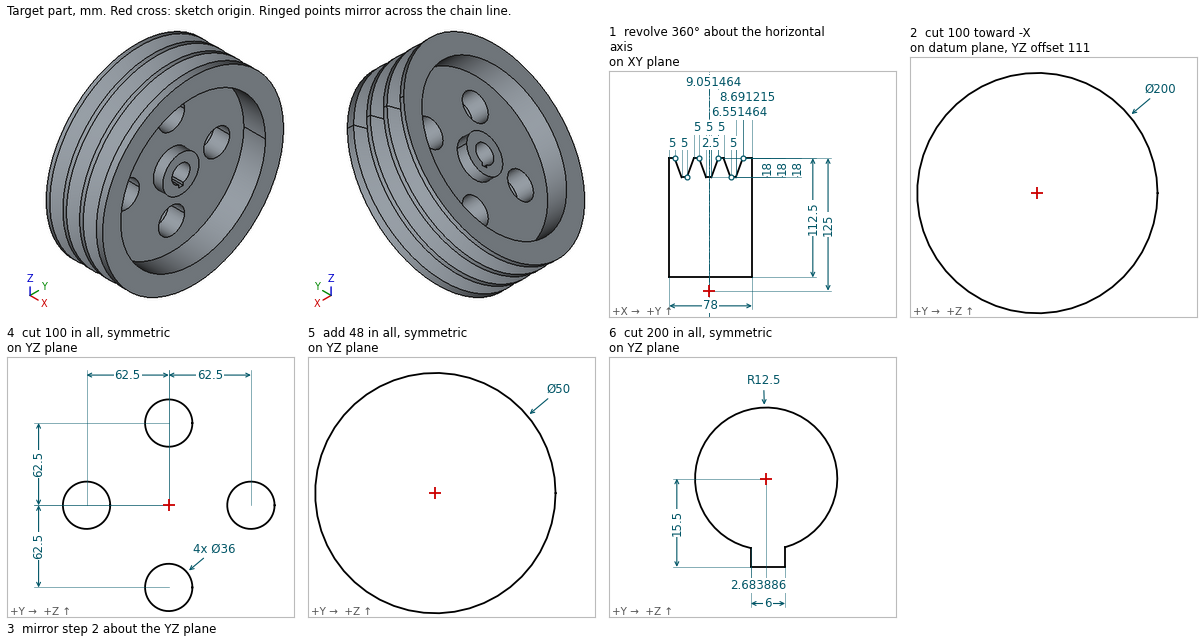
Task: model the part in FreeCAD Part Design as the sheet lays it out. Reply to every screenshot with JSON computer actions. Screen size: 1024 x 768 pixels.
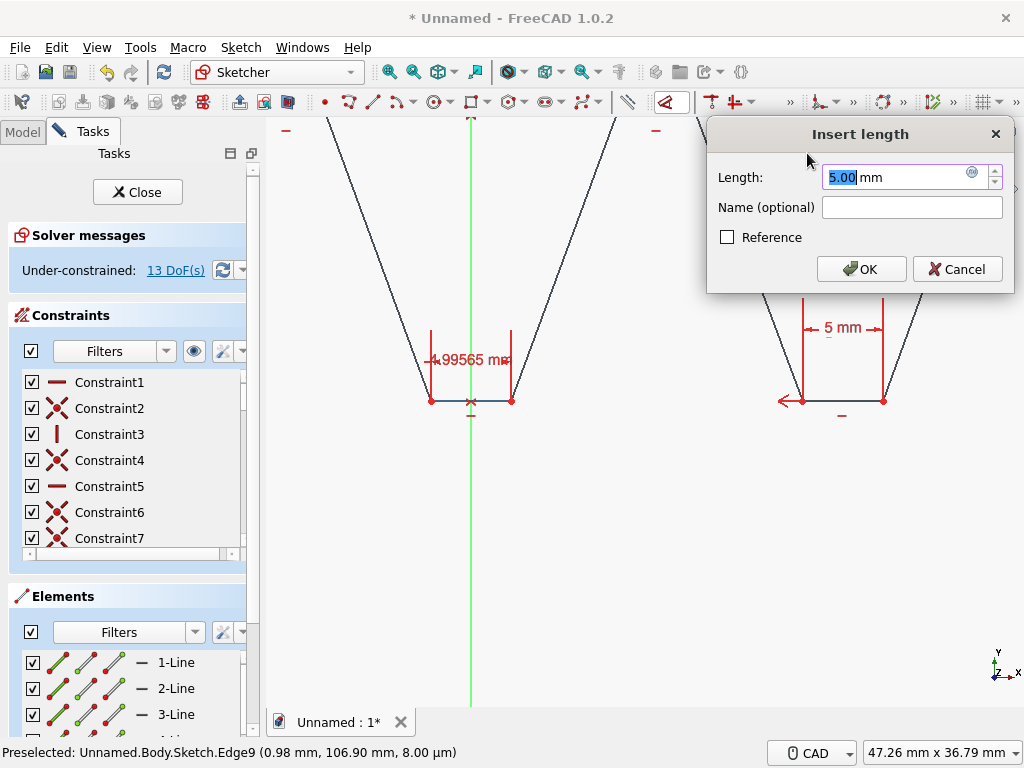
{"action": "type", "text": "5"}
{"action": "key", "text": "Return"}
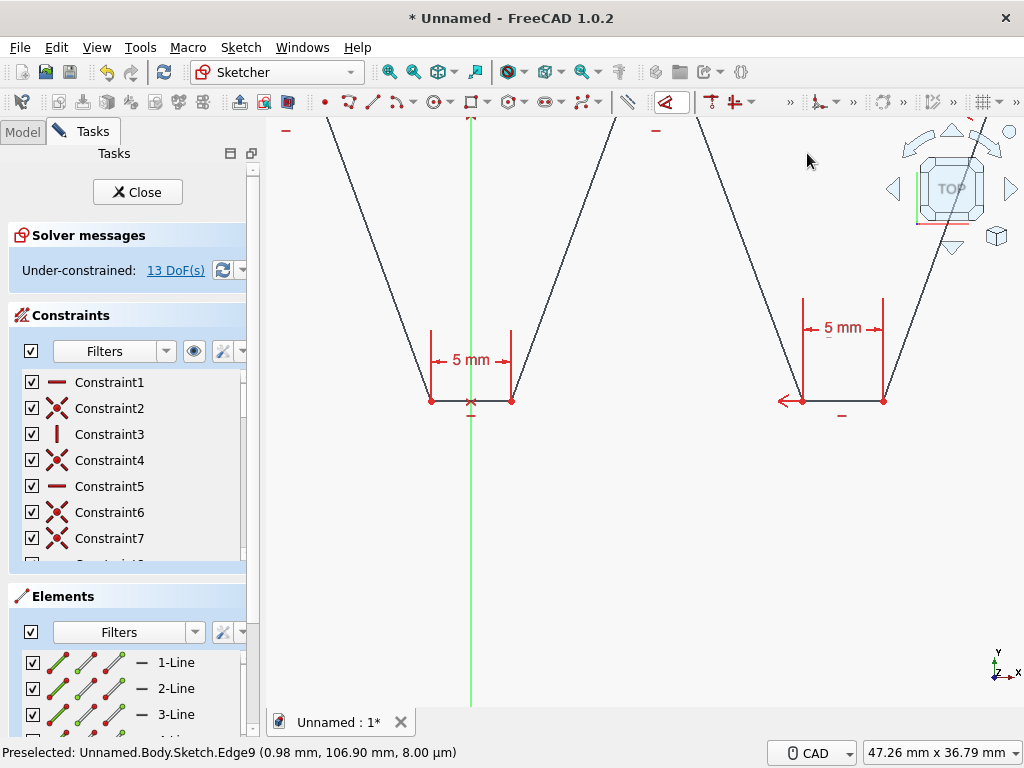
{"action": "scroll", "coordinate": [596, 235], "scroll_direction": "down", "scroll_amount": 8}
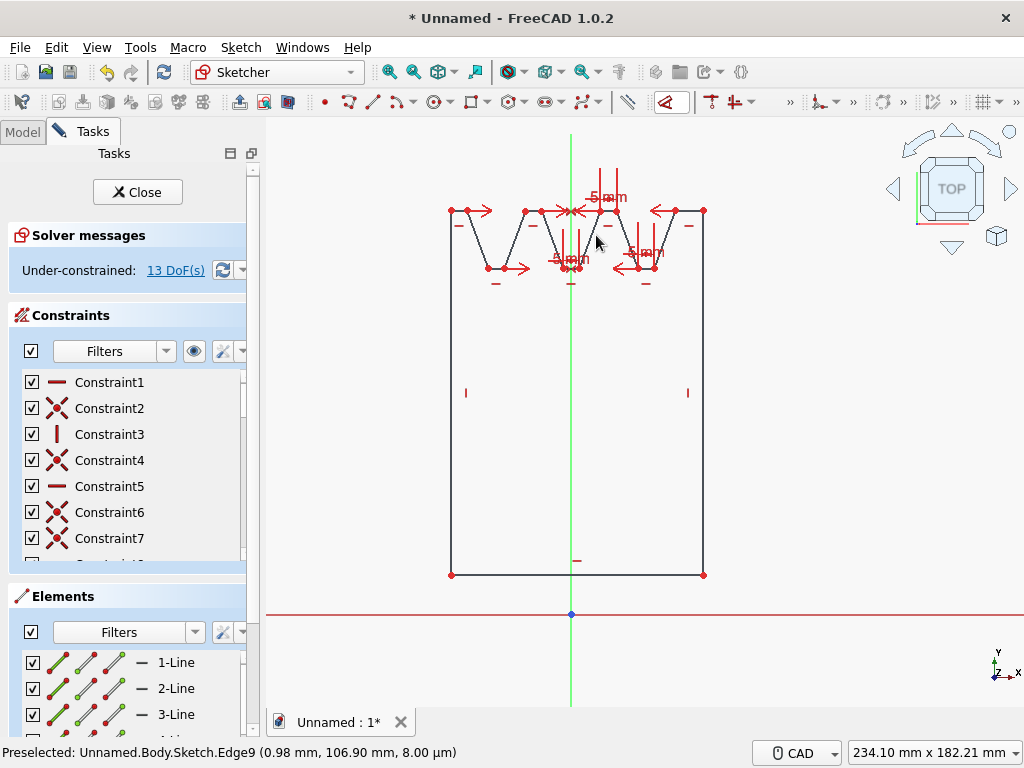
{"action": "scroll", "coordinate": [537, 211], "scroll_direction": "up", "scroll_amount": 6}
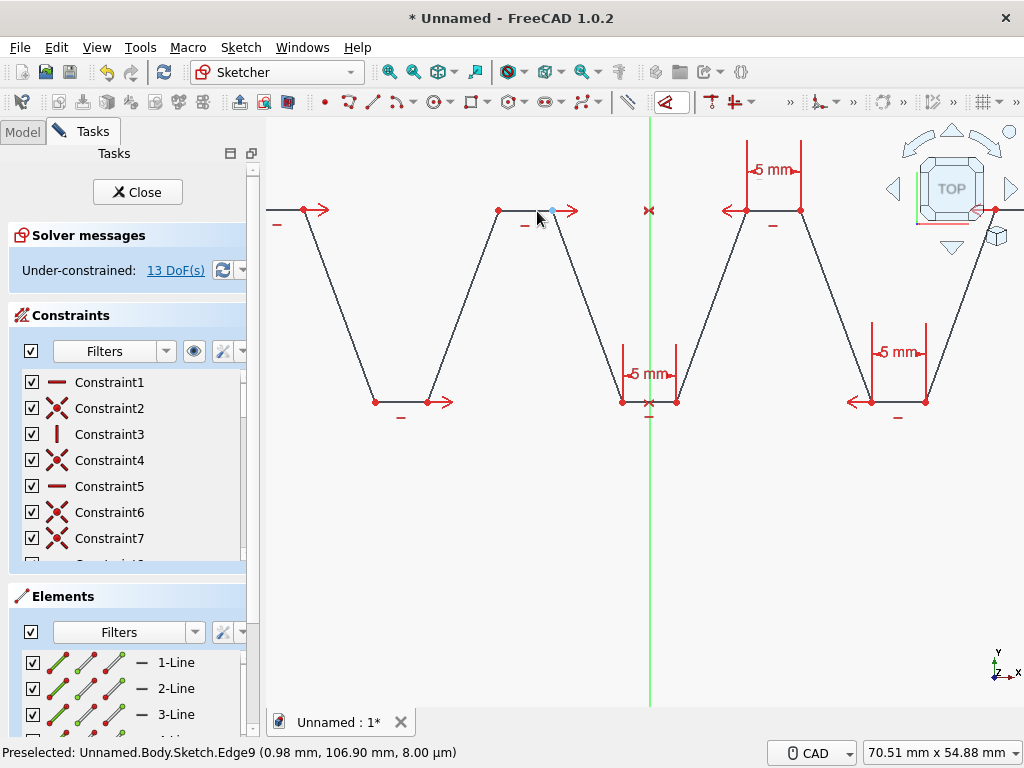
{"action": "left_click", "coordinate": [536, 211]}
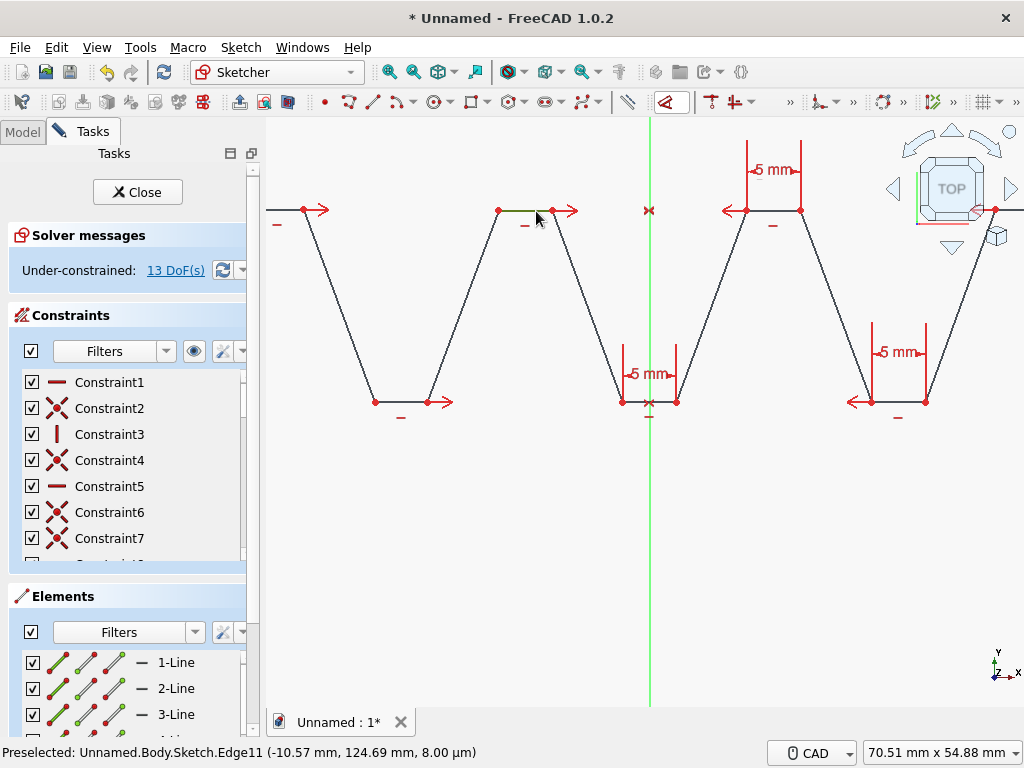
{"action": "left_click", "coordinate": [684, 102]}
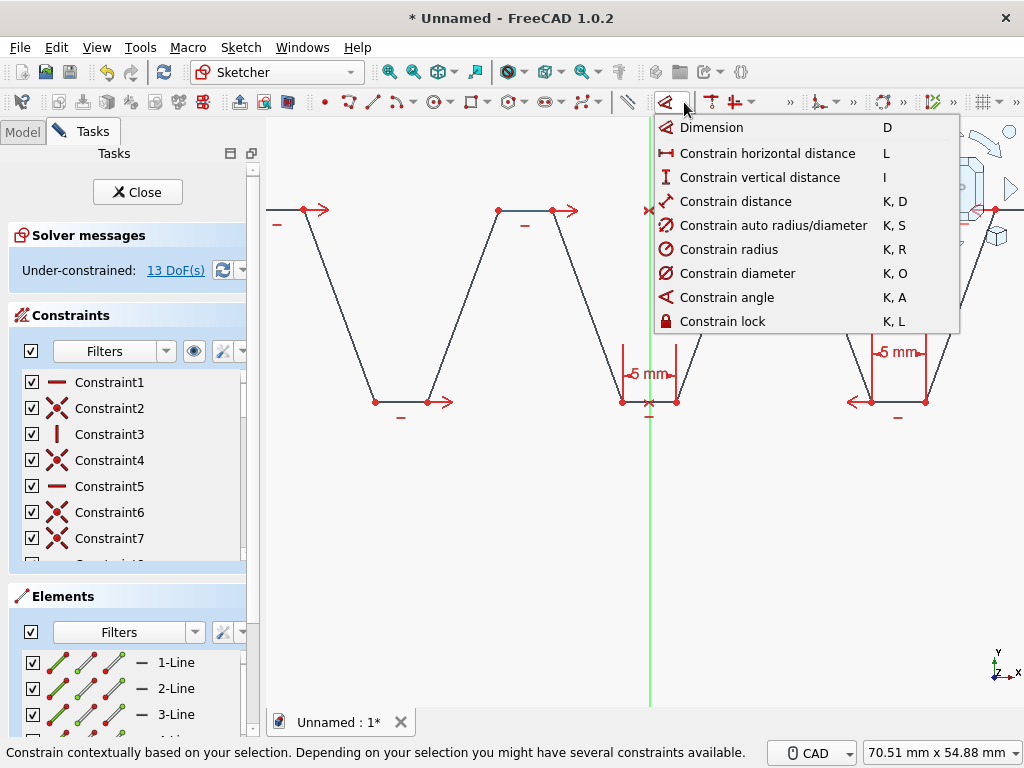
{"action": "left_click", "coordinate": [807, 153]}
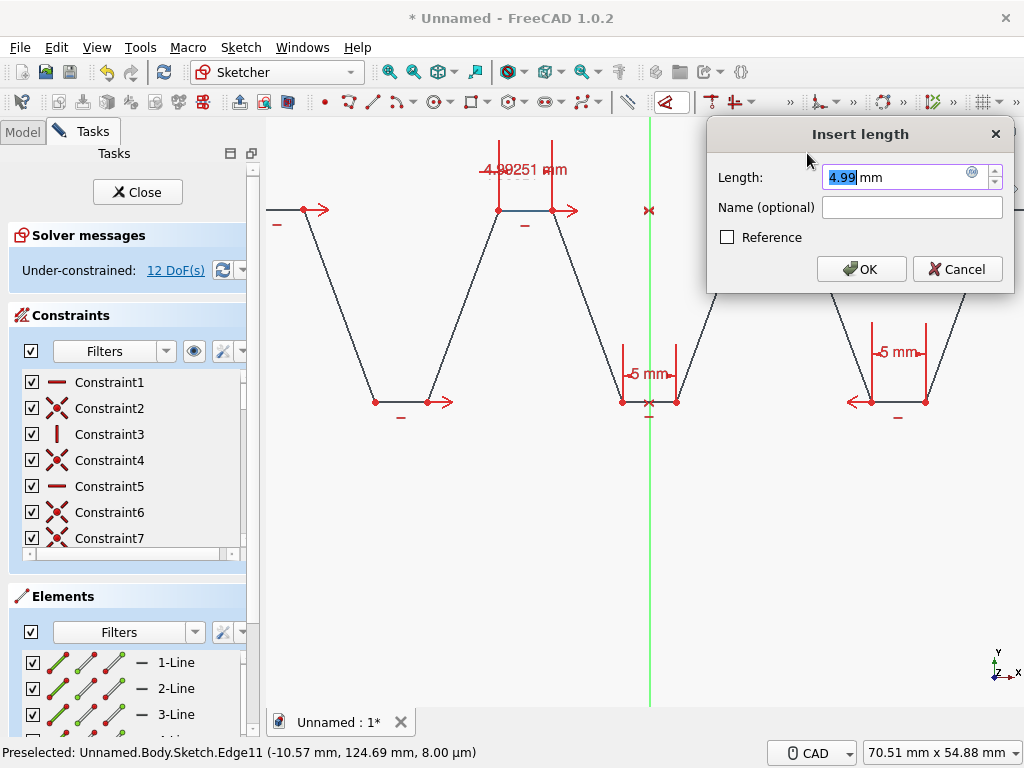
{"action": "type", "text": "5"}
{"action": "key", "text": "Return"}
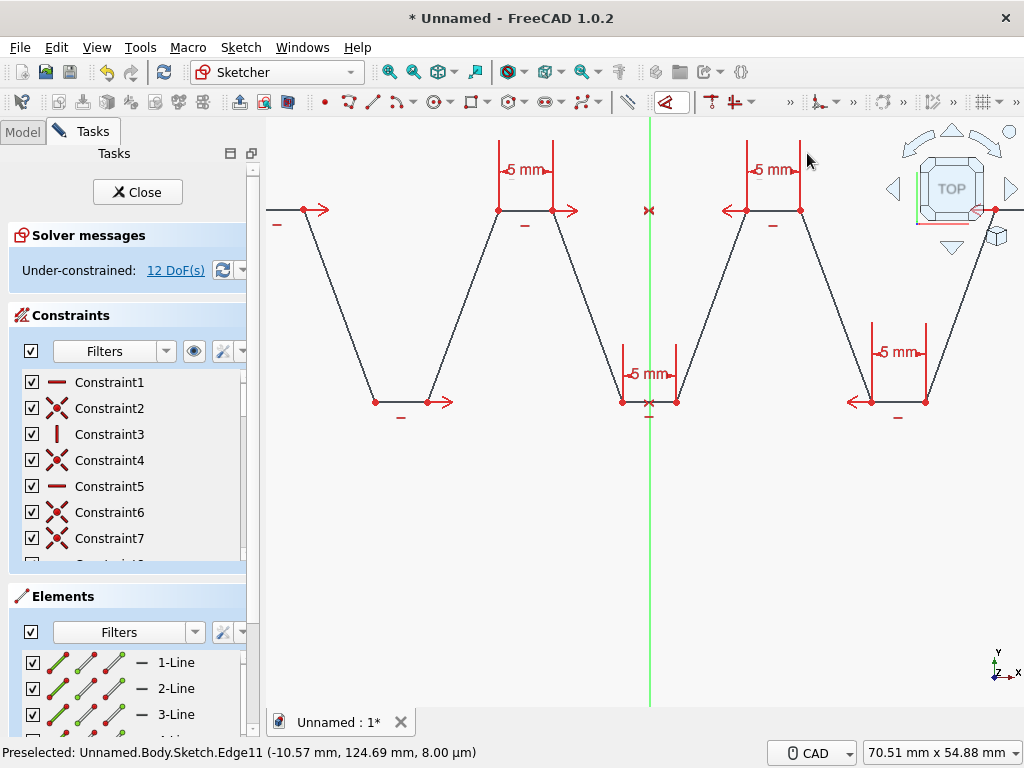
{"action": "left_click", "coordinate": [412, 402]}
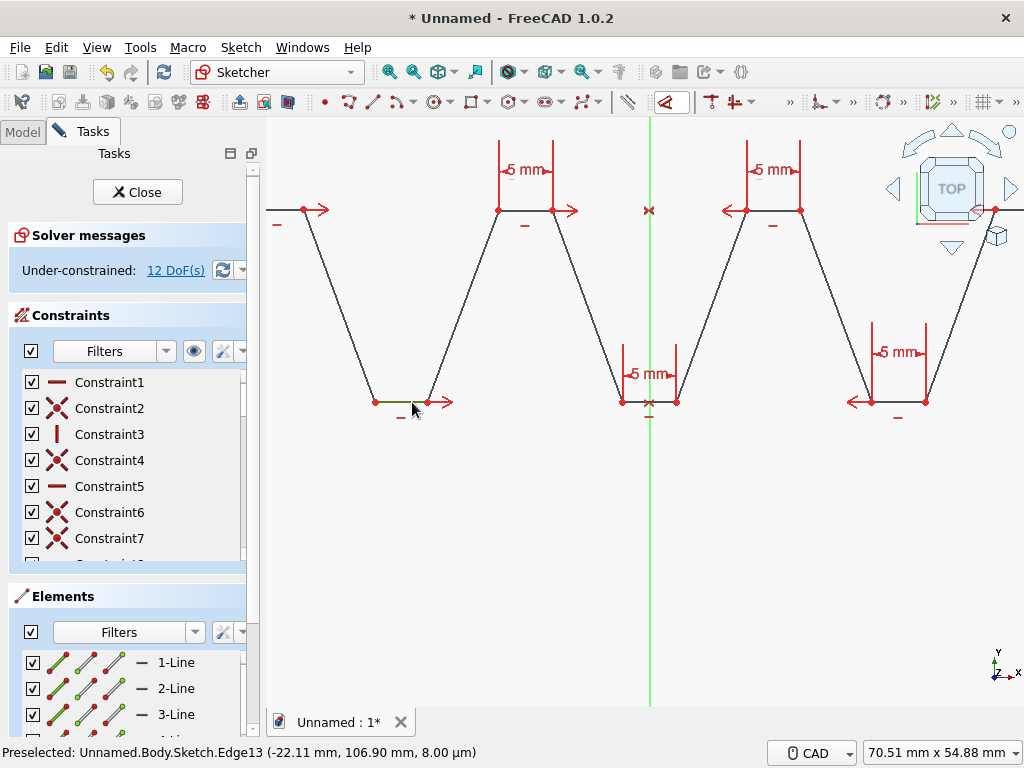
{"action": "key", "text": "l"}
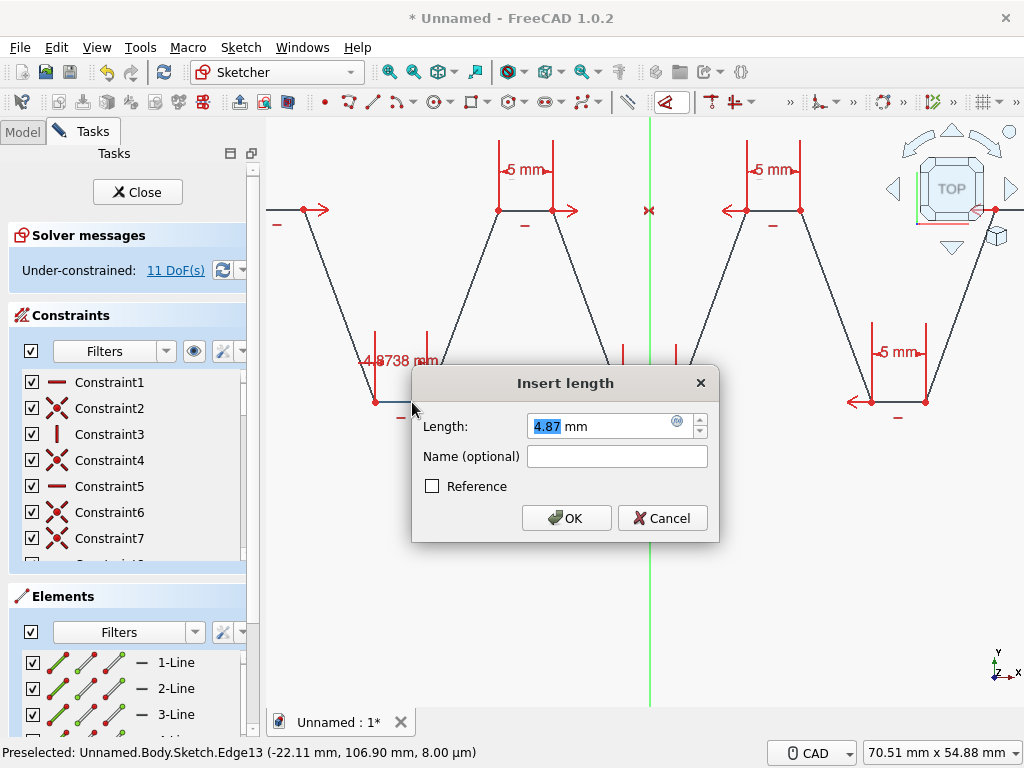
{"action": "type", "text": "5"}
{"action": "key", "text": "Return"}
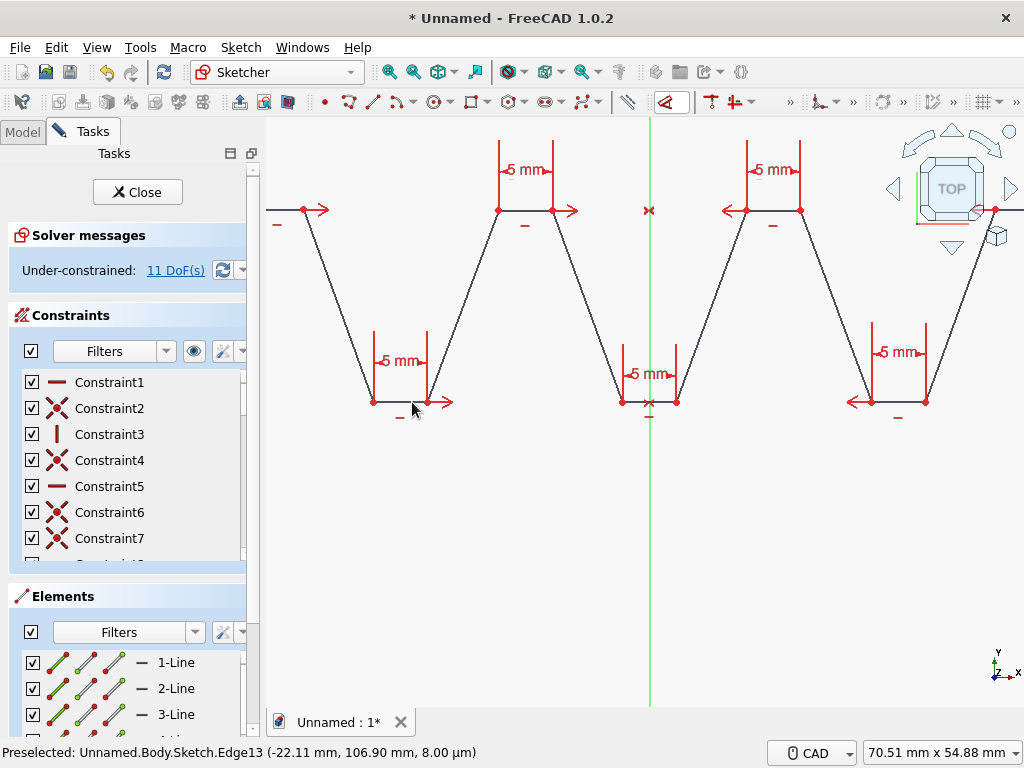
{"action": "scroll", "coordinate": [536, 210], "scroll_direction": "down", "scroll_amount": 6}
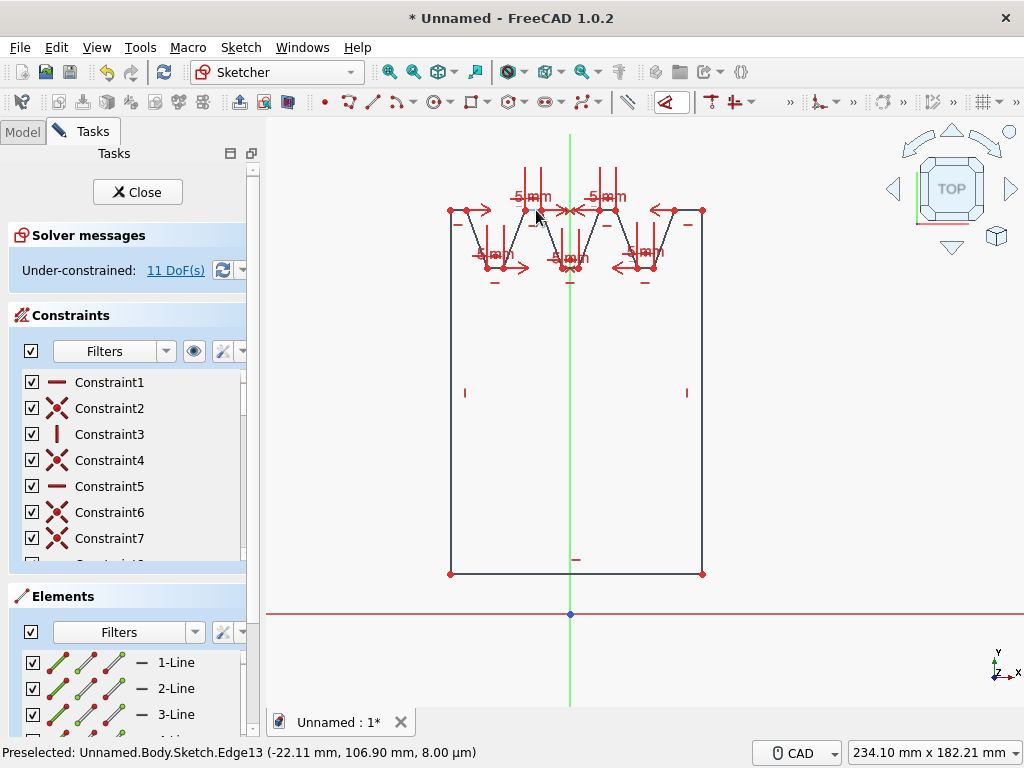
{"action": "scroll", "coordinate": [462, 210], "scroll_direction": "up", "scroll_amount": 6}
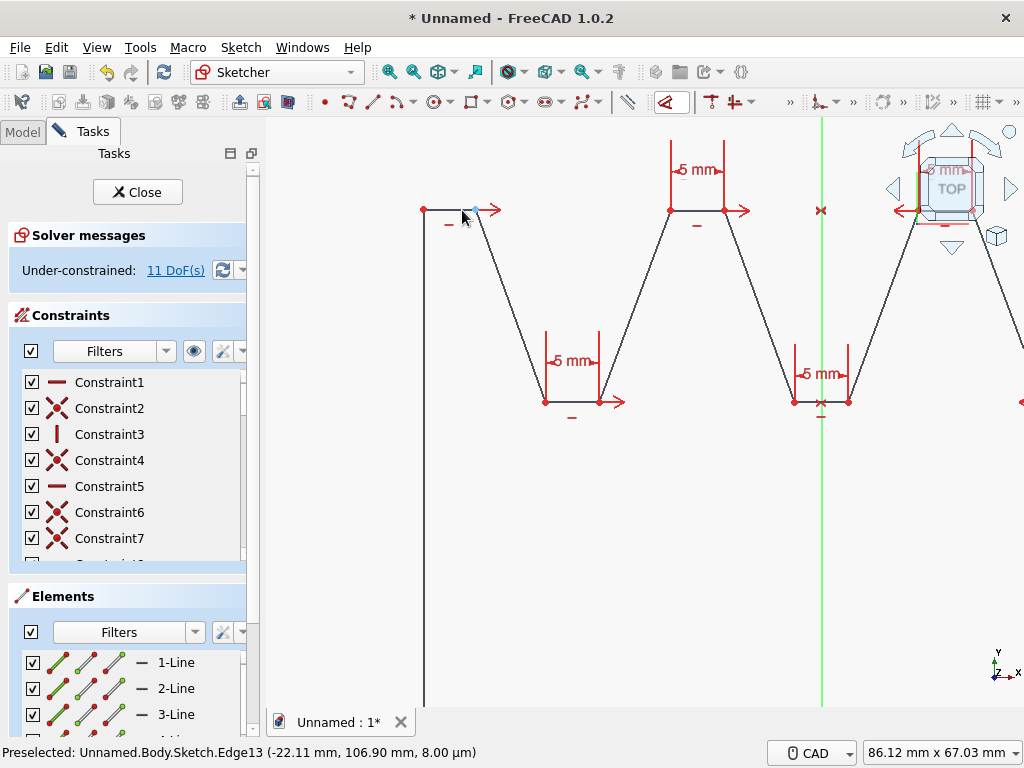
{"action": "left_click", "coordinate": [460, 210]}